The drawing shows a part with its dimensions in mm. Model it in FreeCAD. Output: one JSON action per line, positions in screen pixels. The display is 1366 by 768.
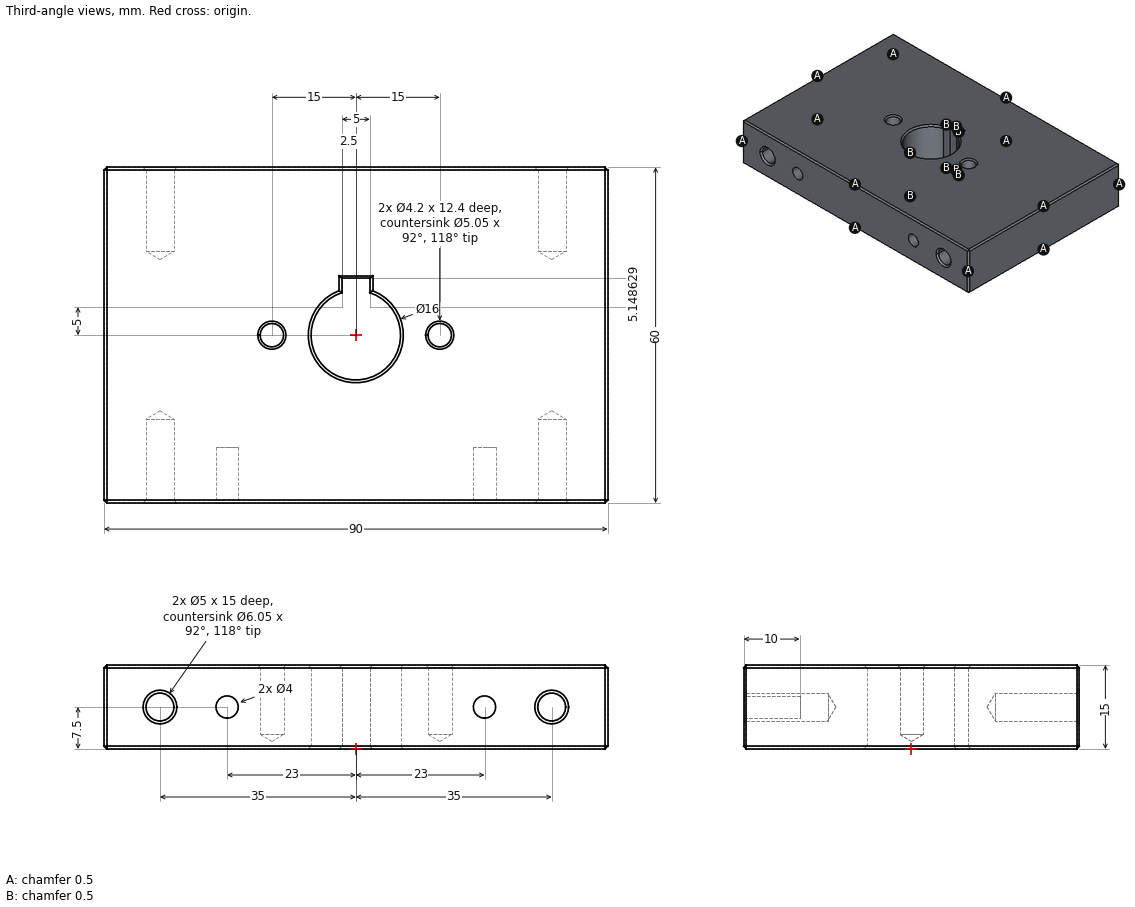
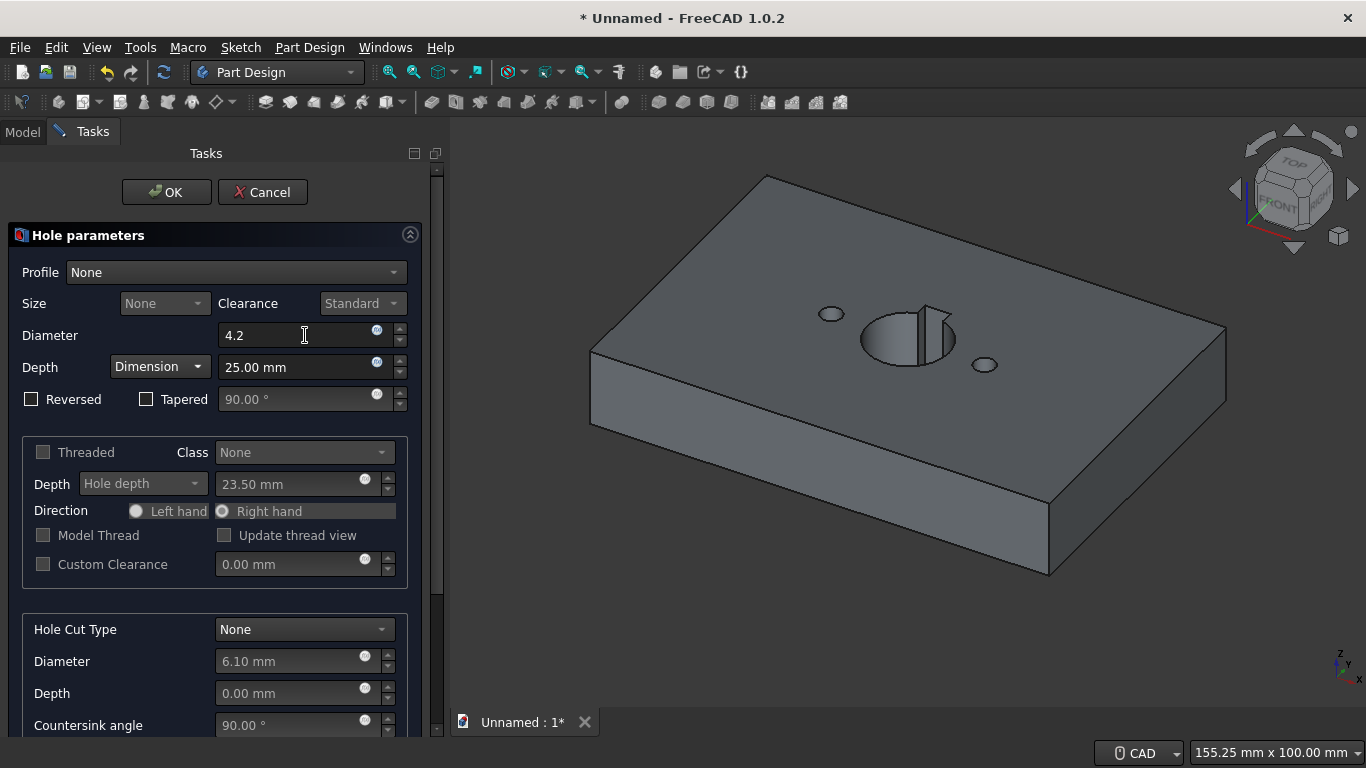
{"action": "triple_click", "coordinate": [305, 367]}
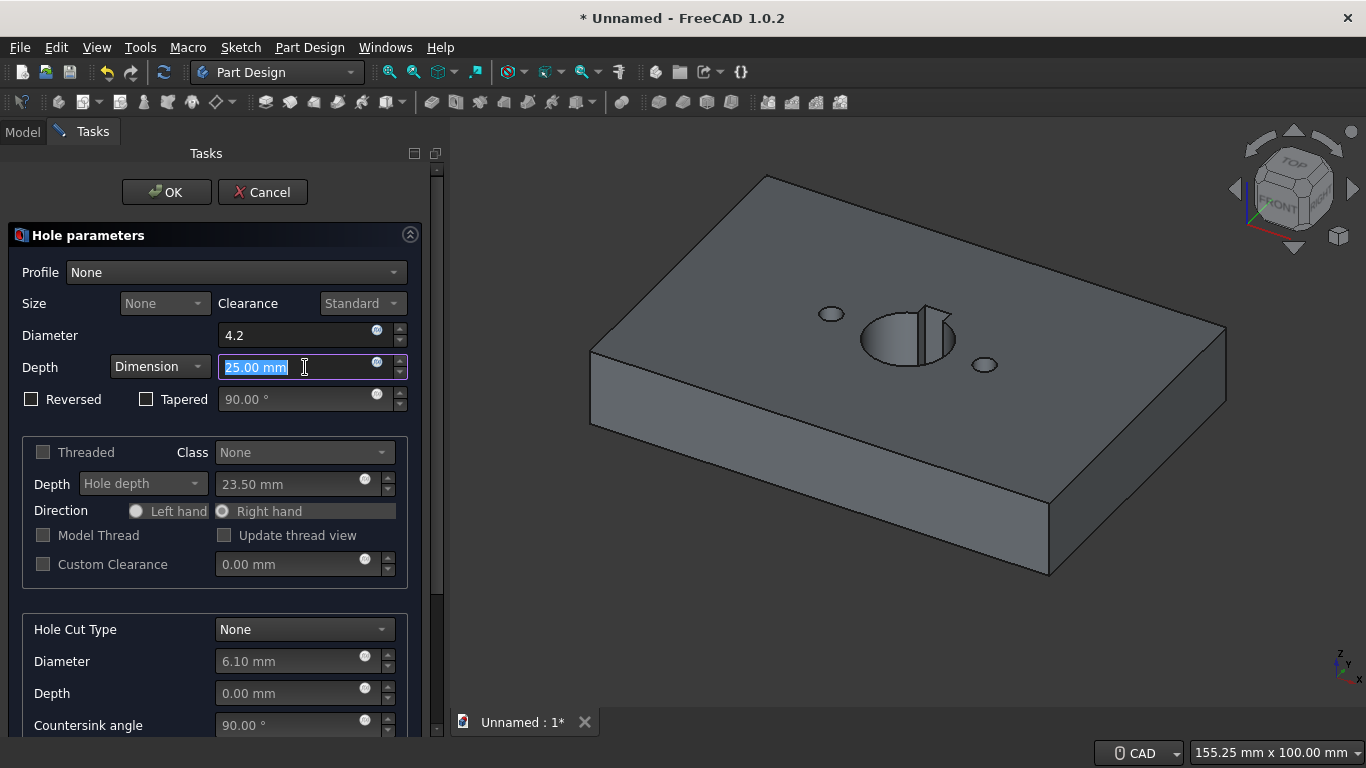
{"action": "type", "text": "12.4"}
{"action": "key", "text": "Tab"}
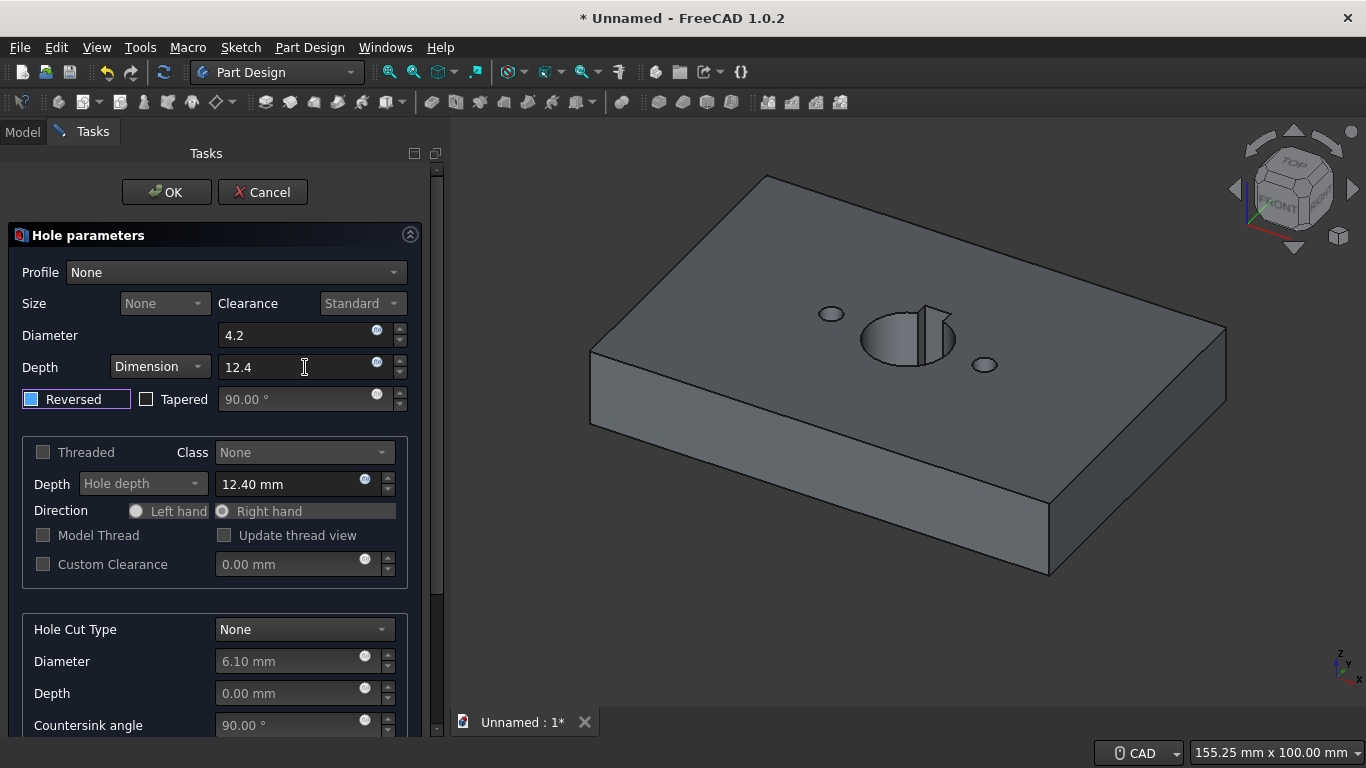
{"action": "left_click", "coordinate": [306, 630]}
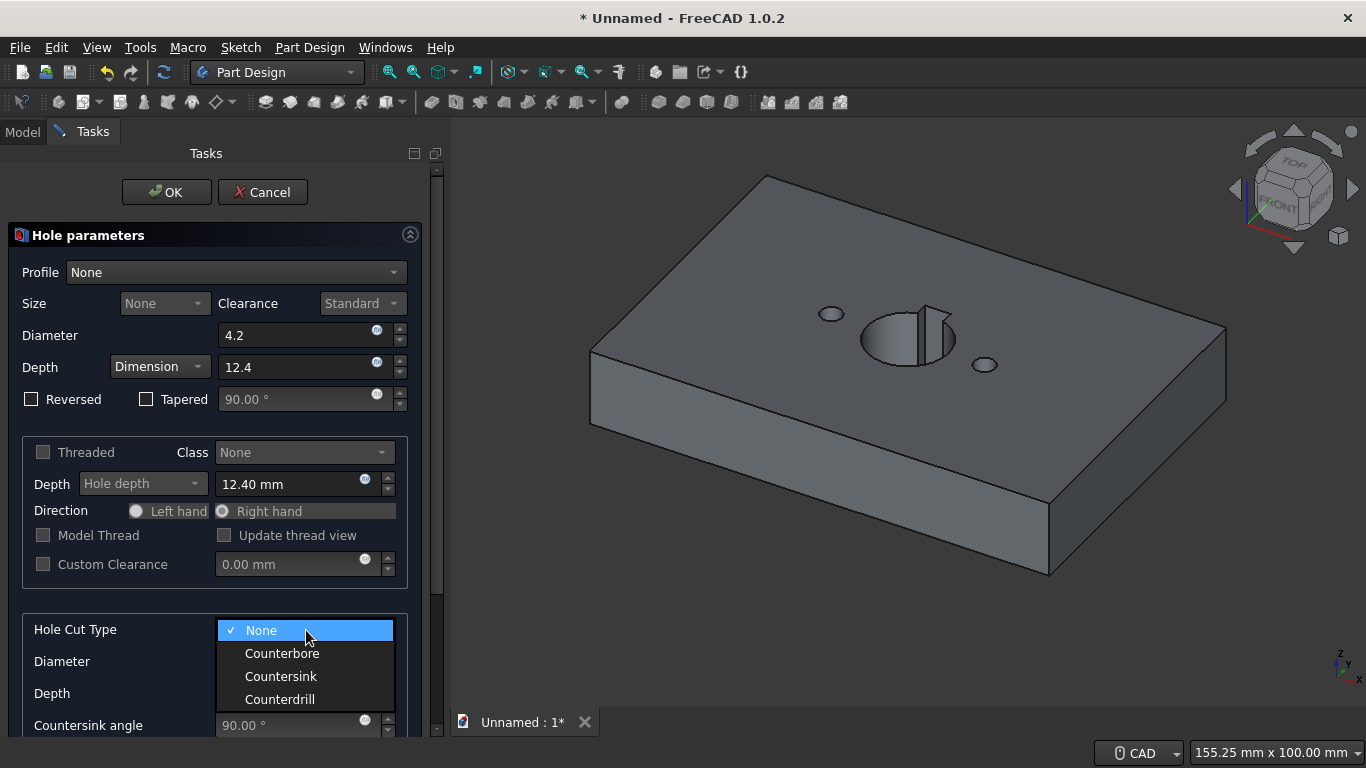
{"action": "left_click", "coordinate": [304, 676]}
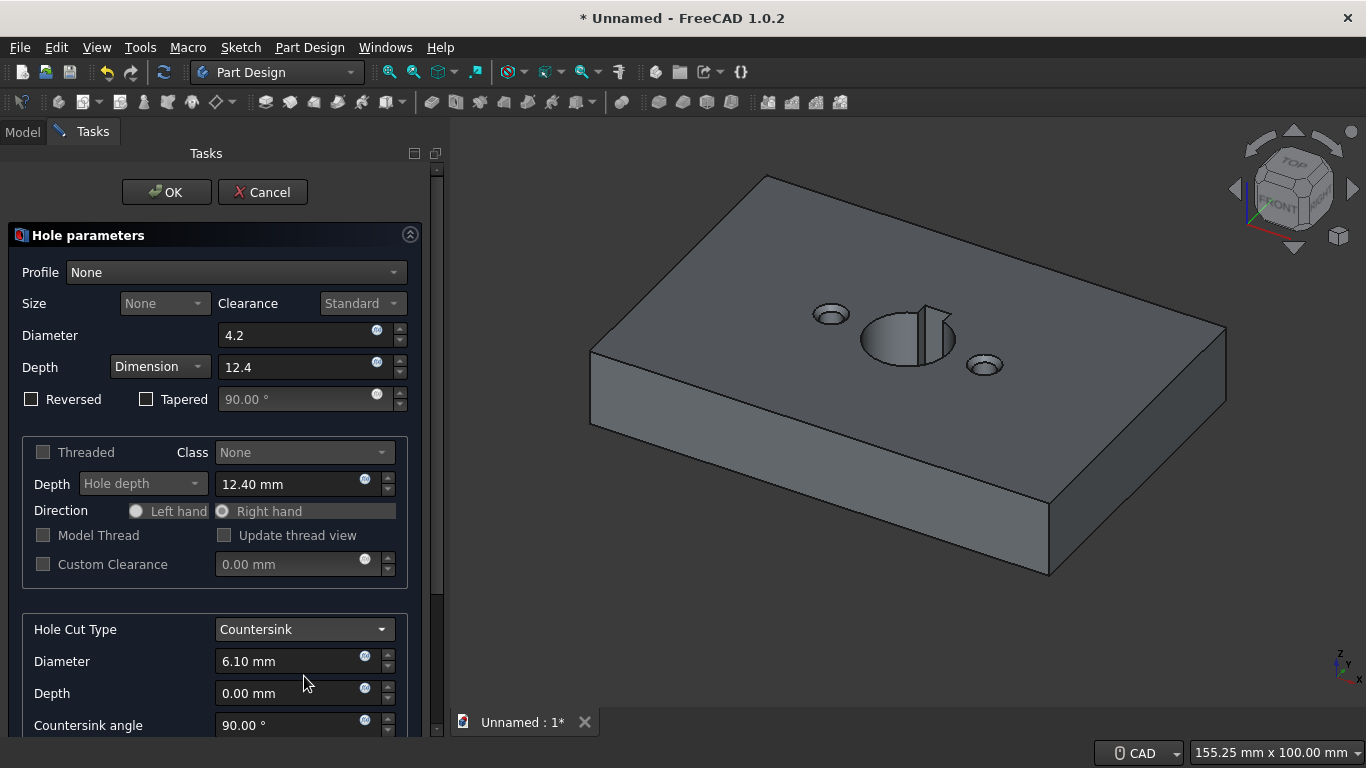
{"action": "scroll", "coordinate": [437, 450], "scroll_direction": "down", "scroll_amount": 2}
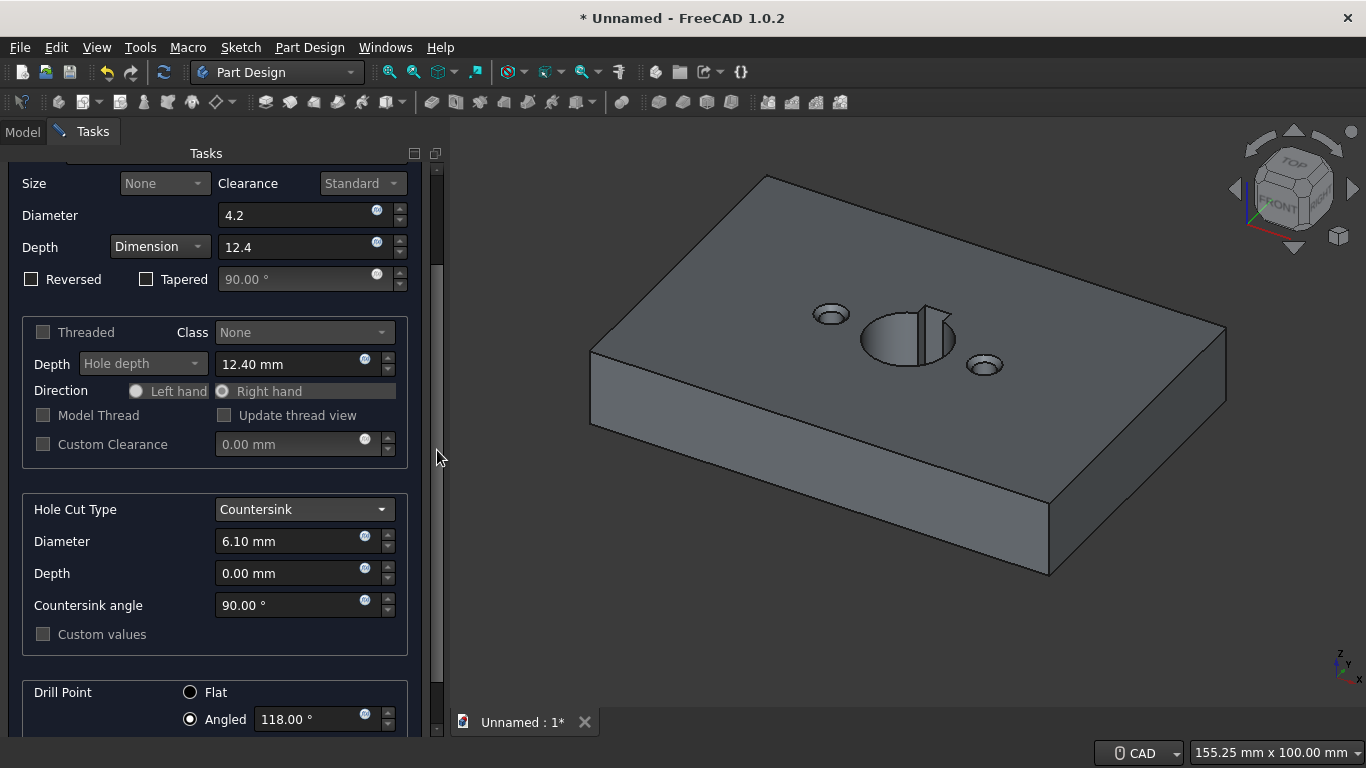
{"action": "triple_click", "coordinate": [298, 605]}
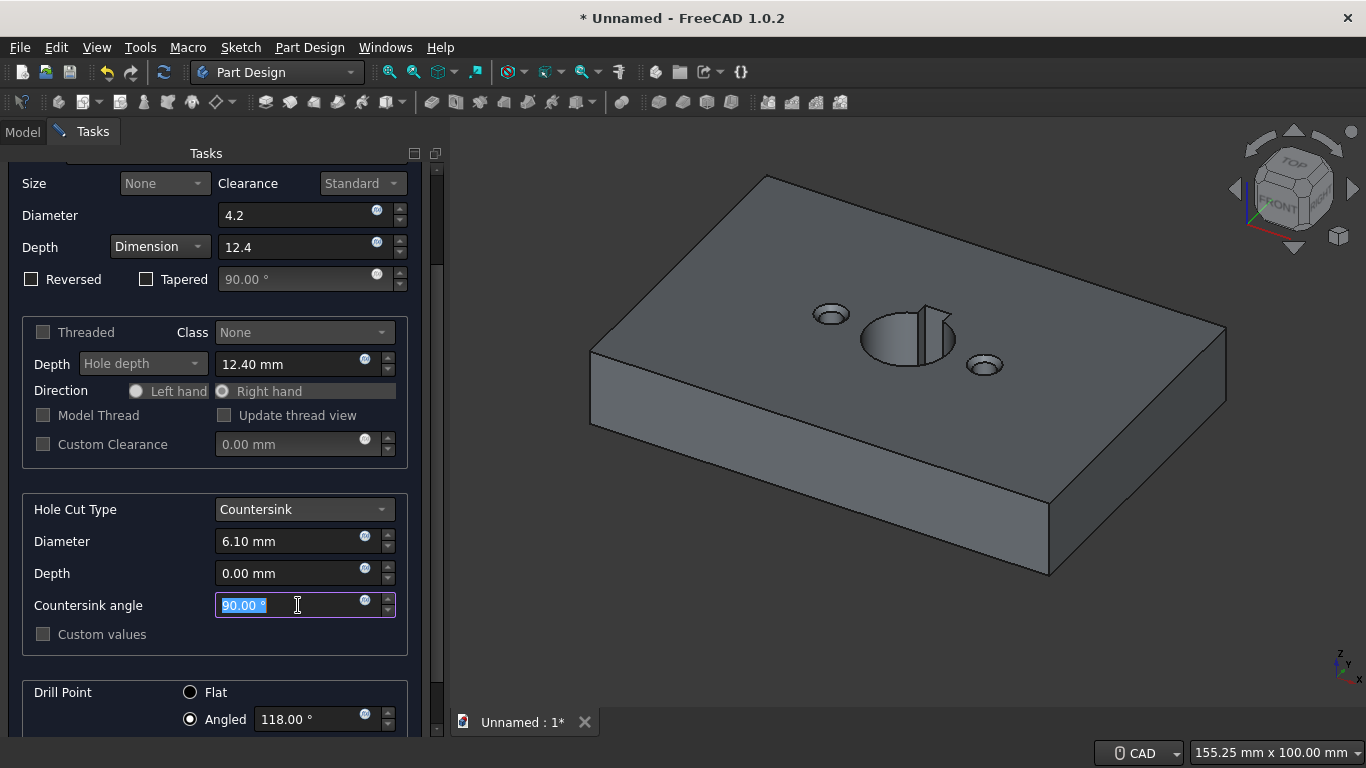
{"action": "type", "text": "92"}
{"action": "key", "text": "Tab"}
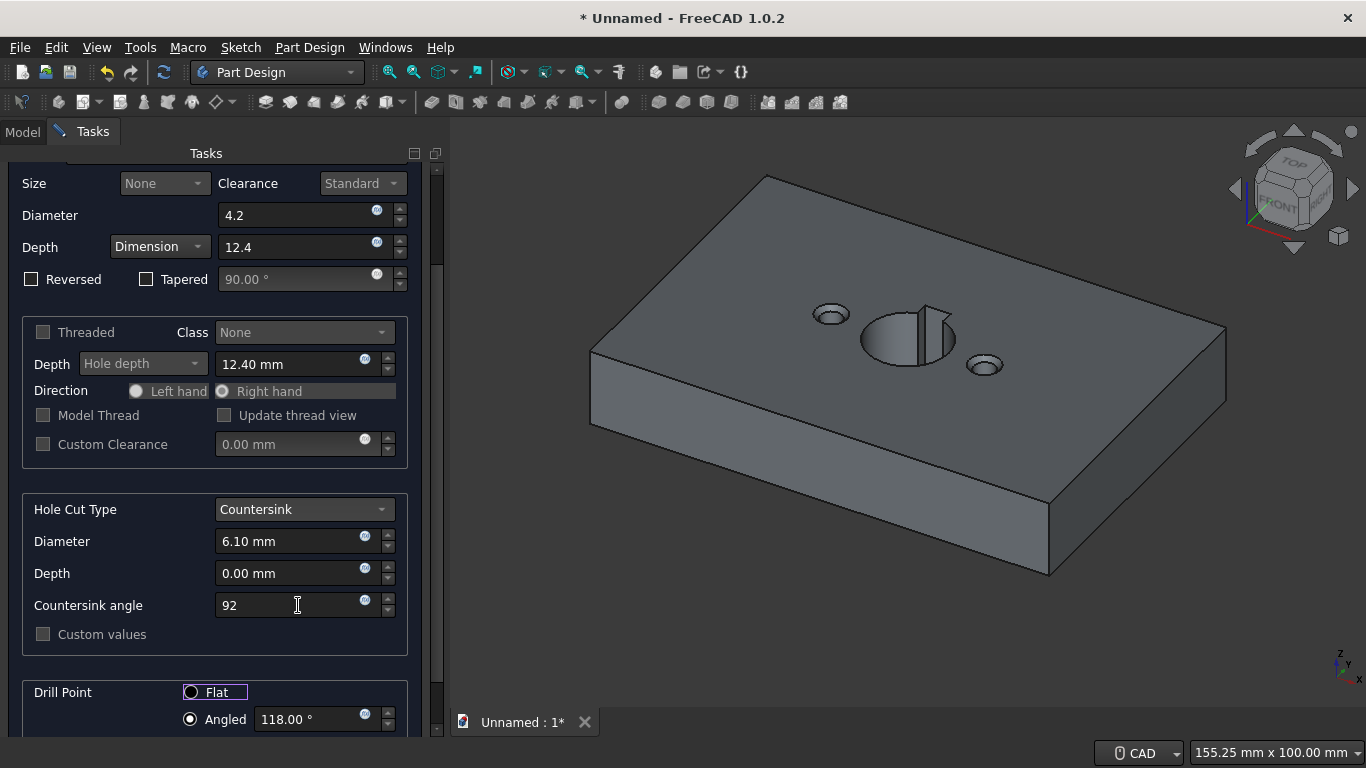
{"action": "triple_click", "coordinate": [298, 541]}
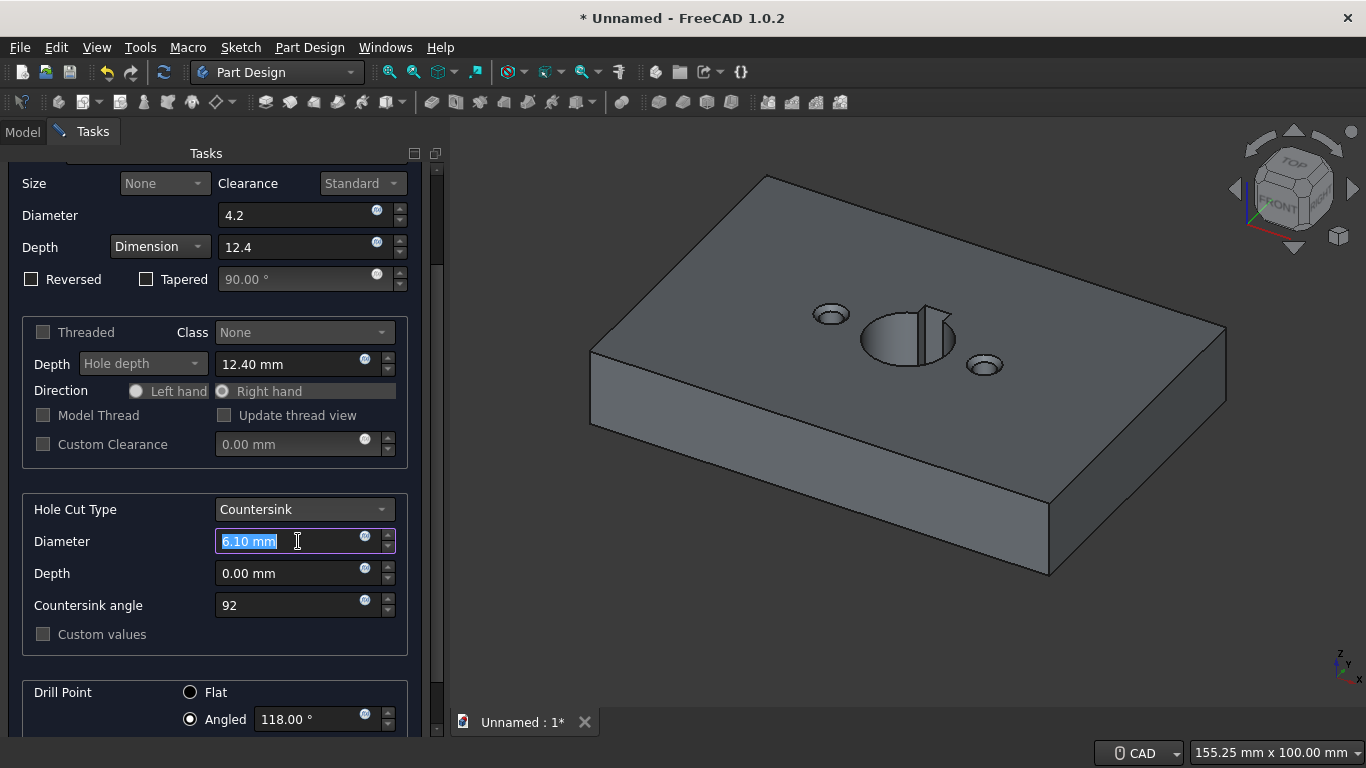
{"action": "type", "text": "5.05"}
{"action": "key", "text": "Tab"}